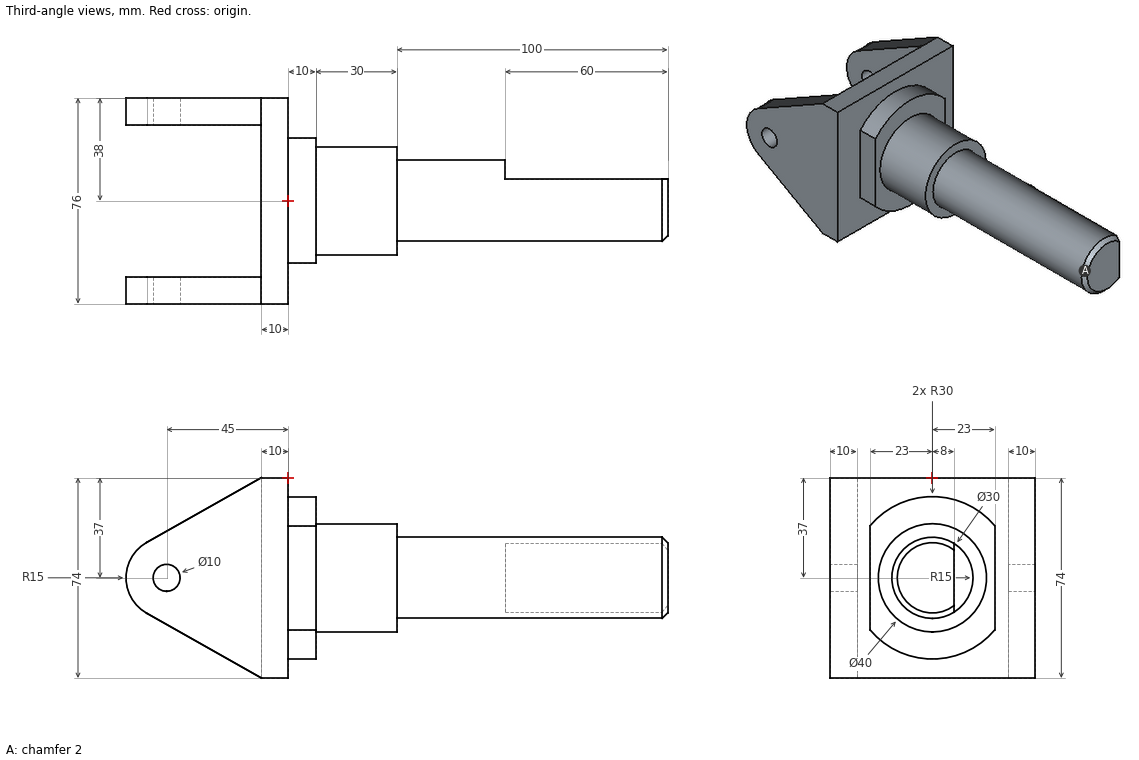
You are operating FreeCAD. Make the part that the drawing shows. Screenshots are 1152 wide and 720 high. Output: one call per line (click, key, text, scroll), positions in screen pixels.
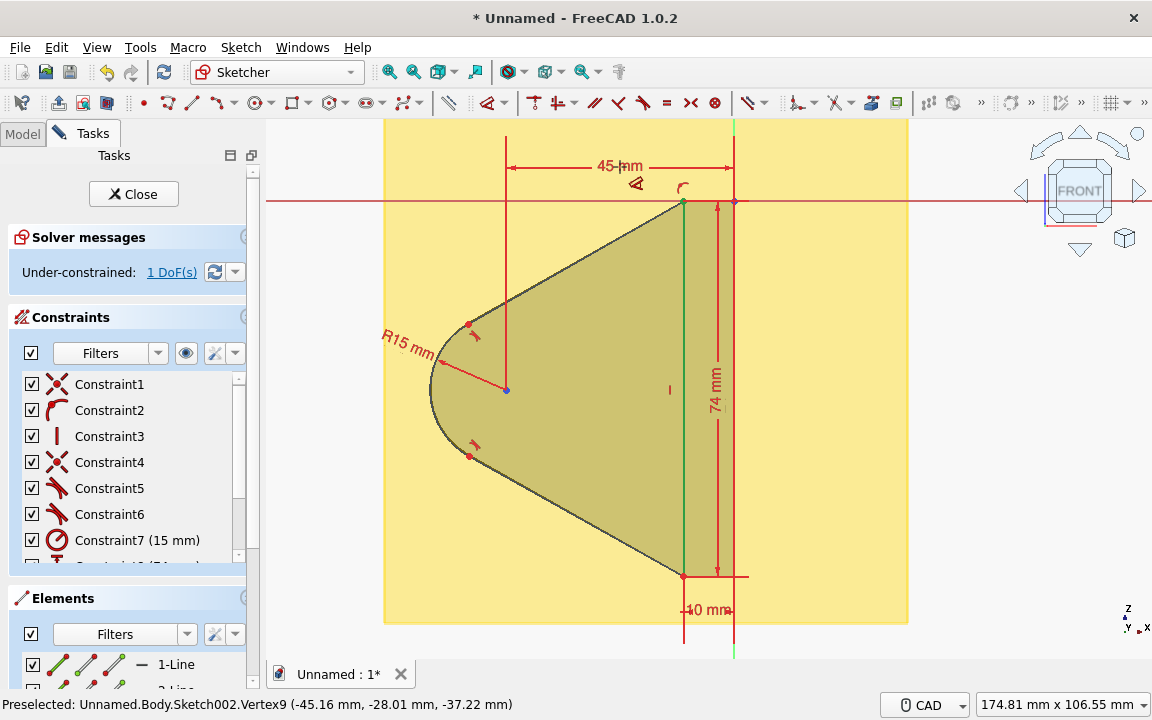
click(506, 390)
click(768, 296)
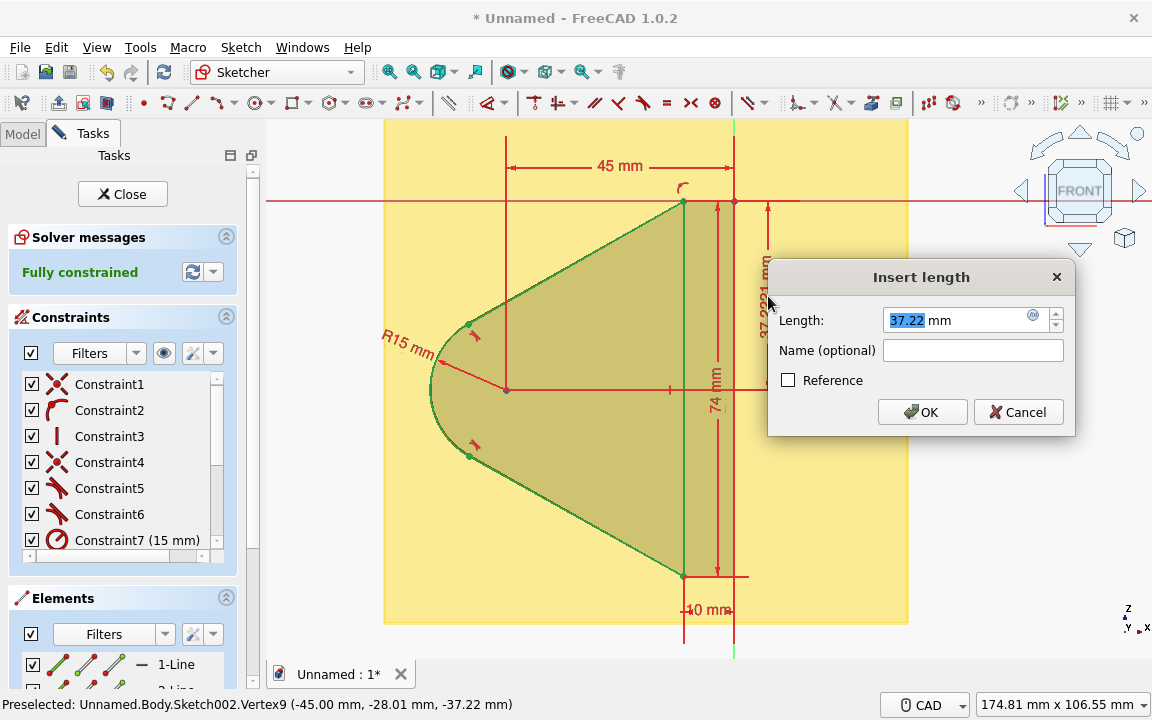
text(37)
key(Return)
key(Escape)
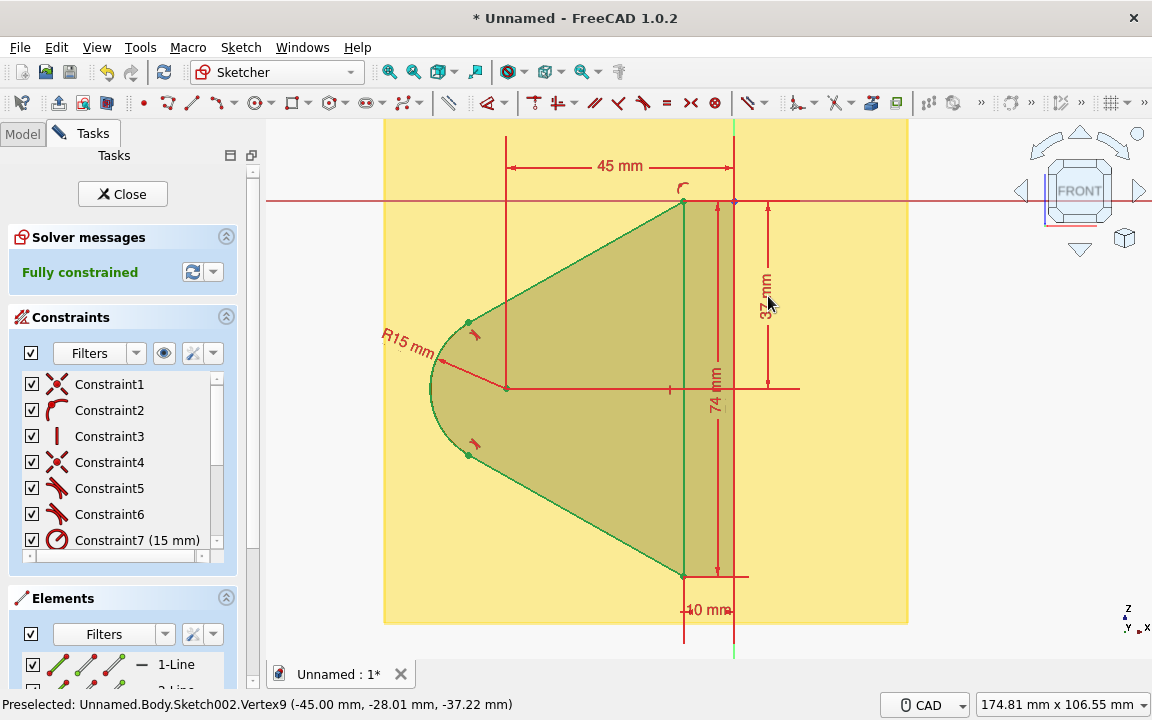
click(123, 194)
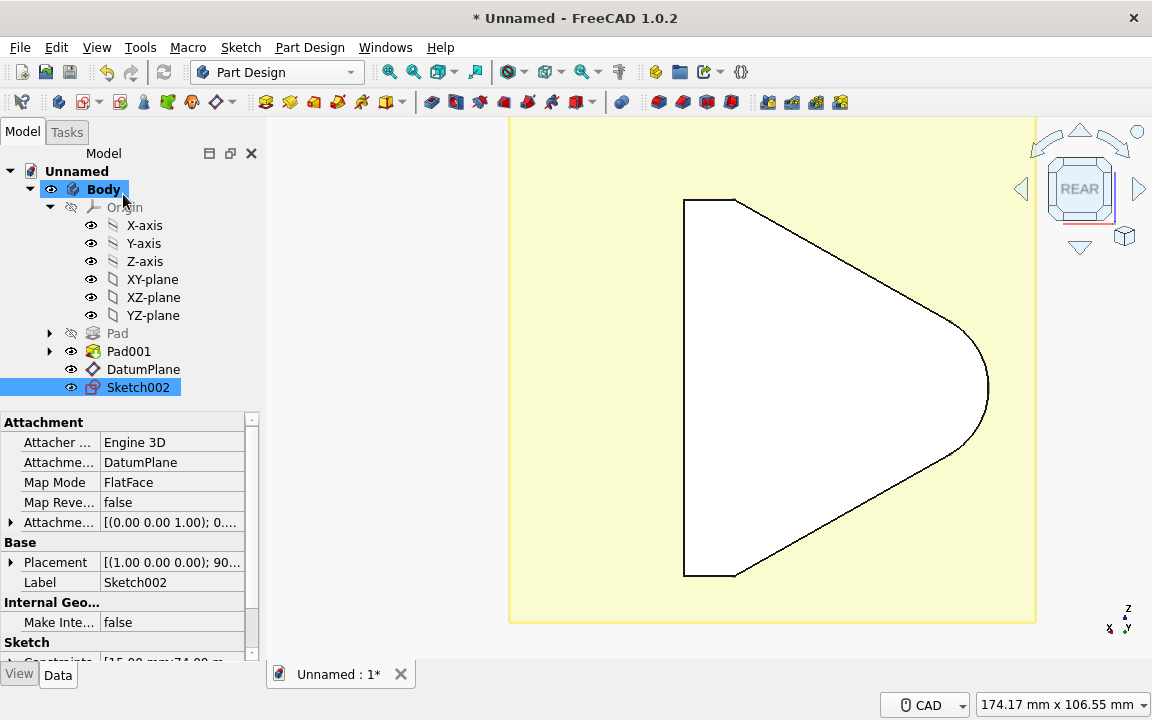
click(266, 102)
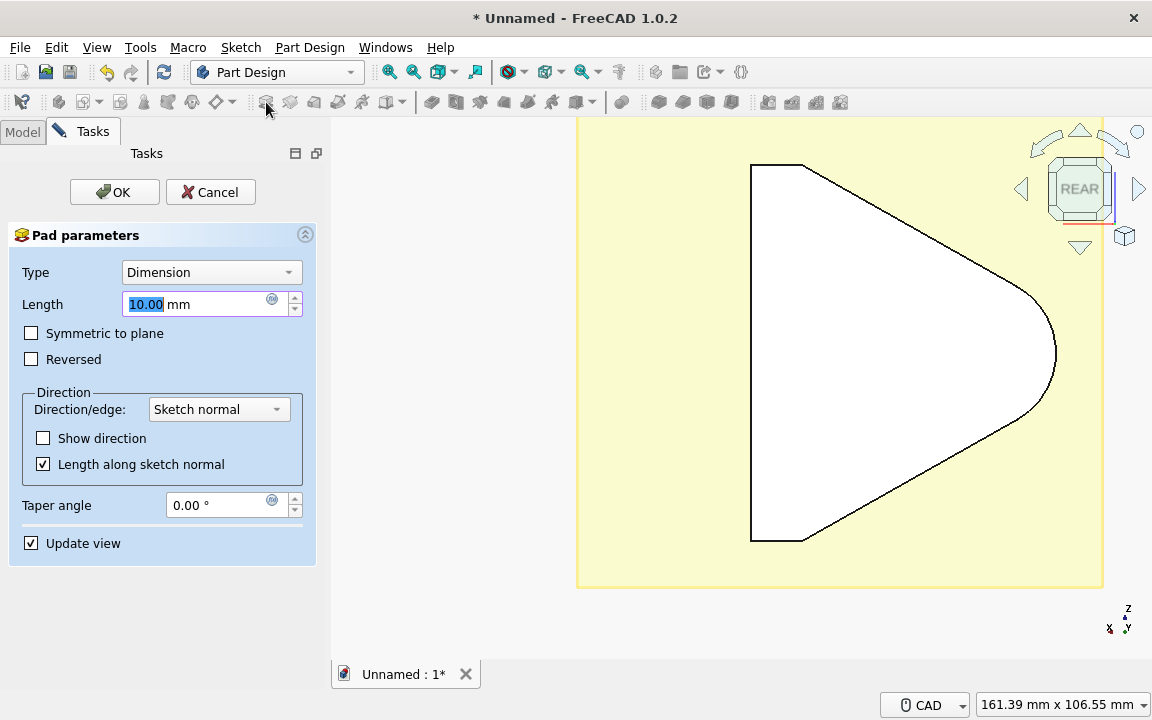
text(10)
key(Tab)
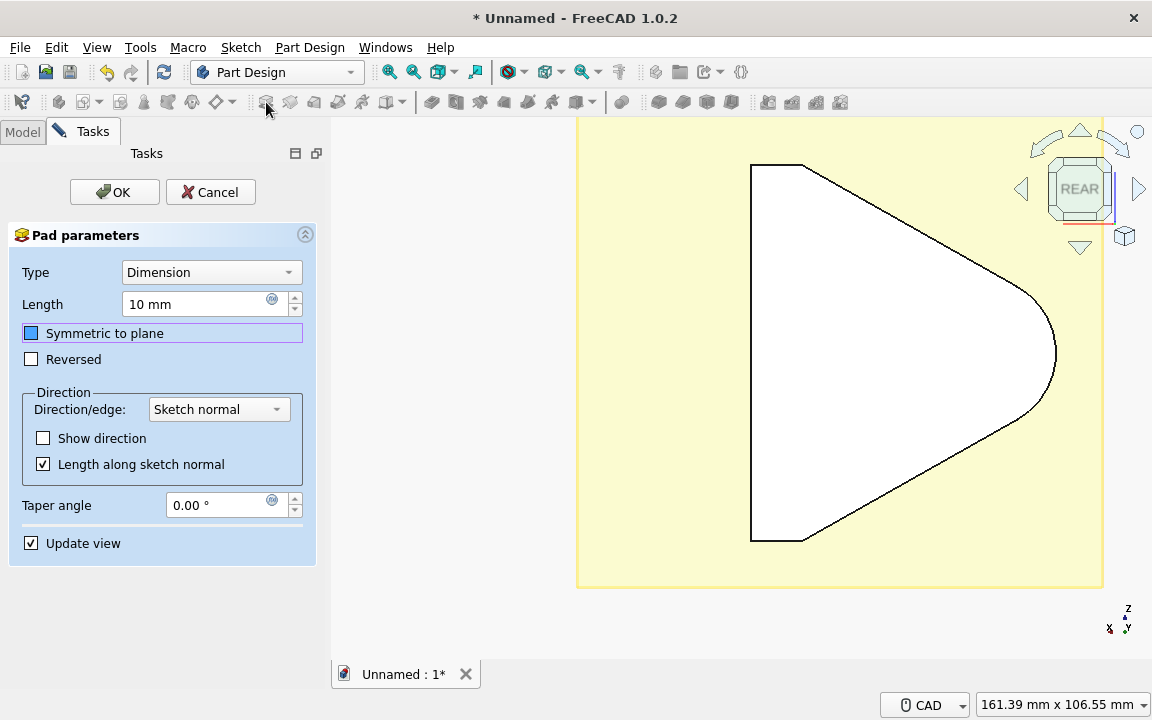
click(115, 192)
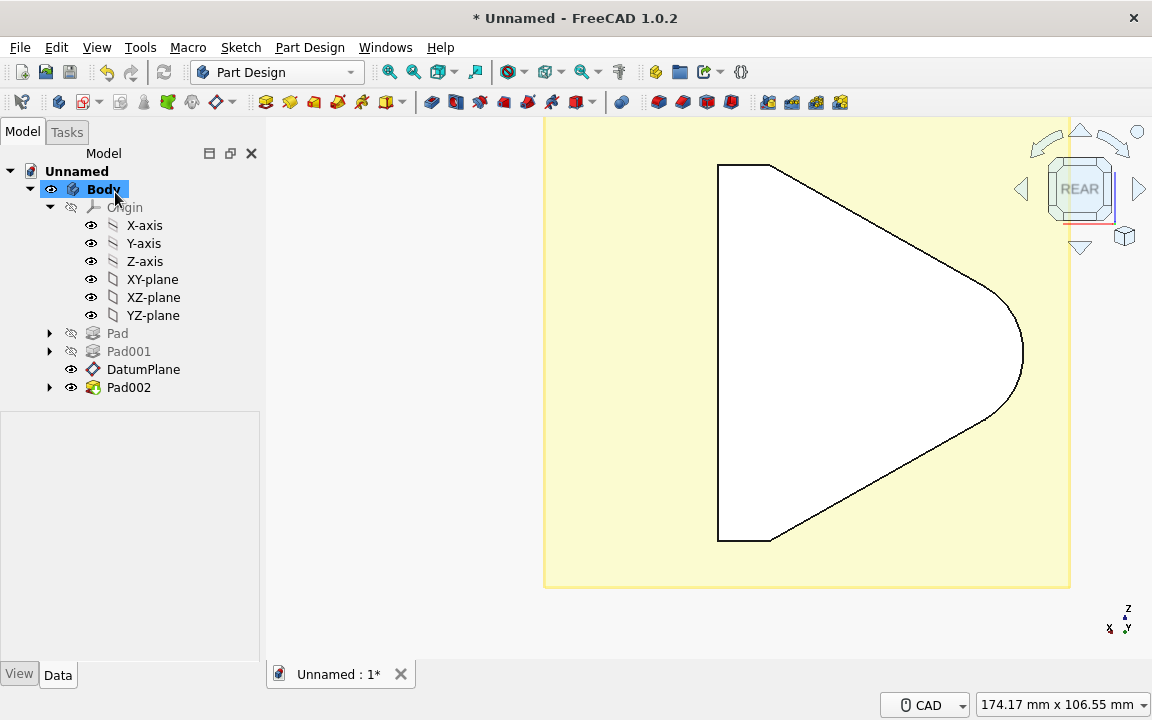
click(116, 369)
key(space)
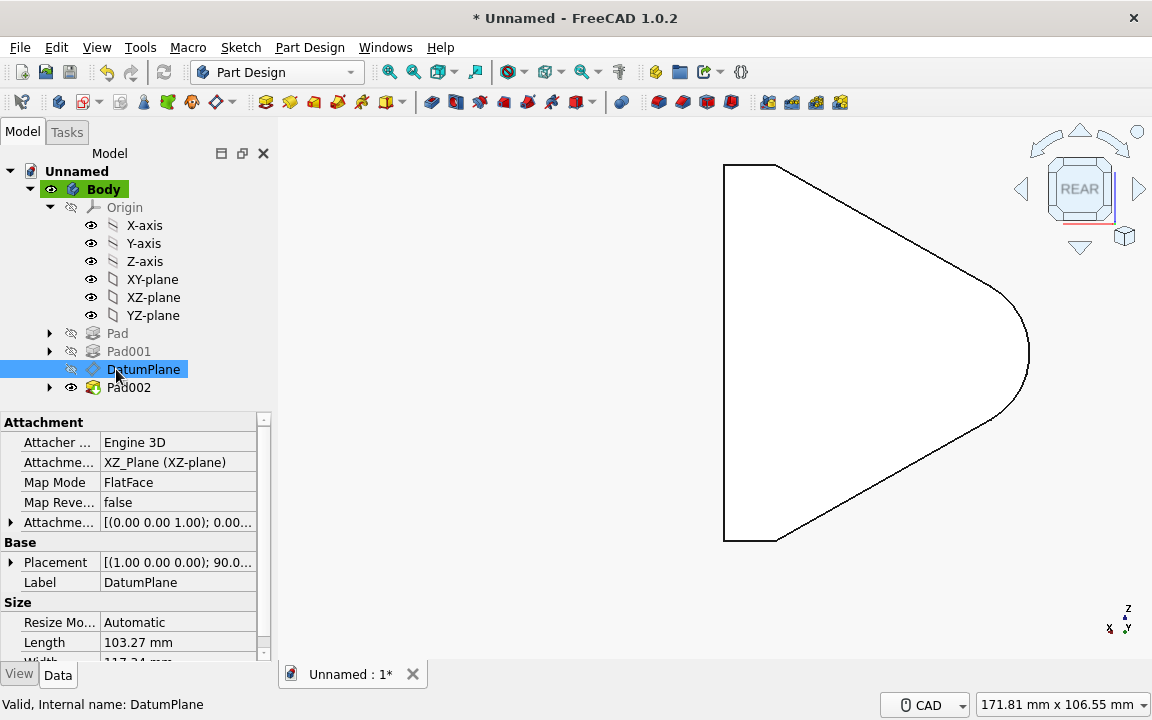
key(0)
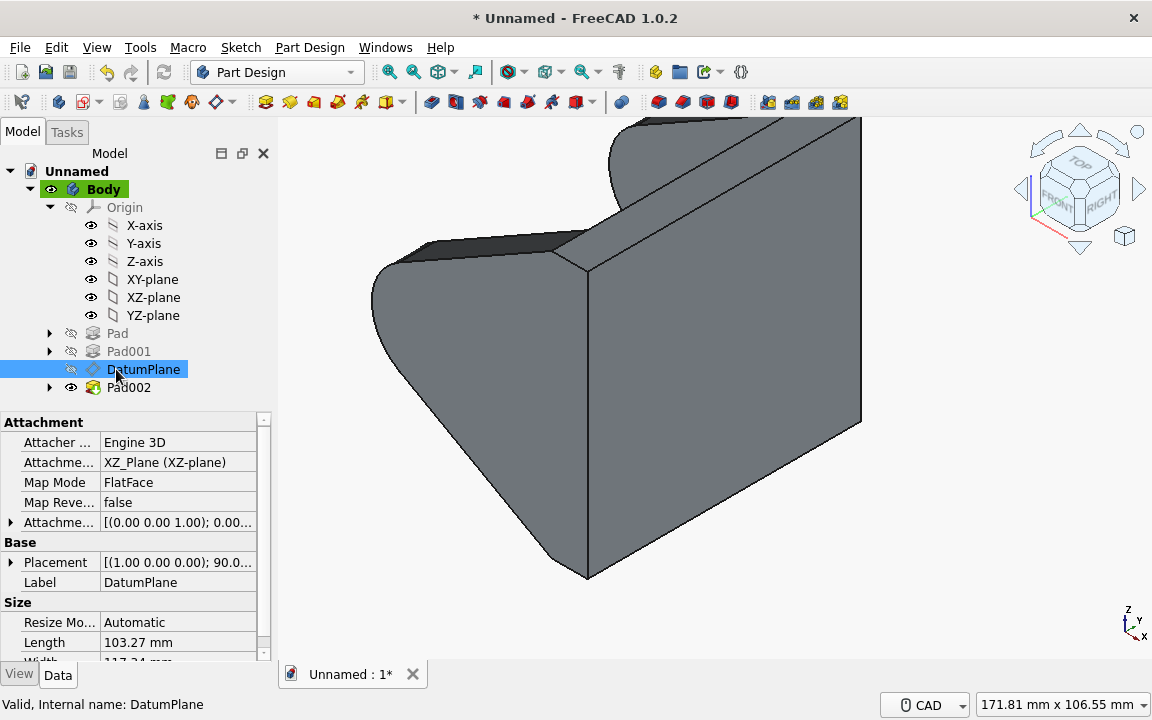
click(390, 72)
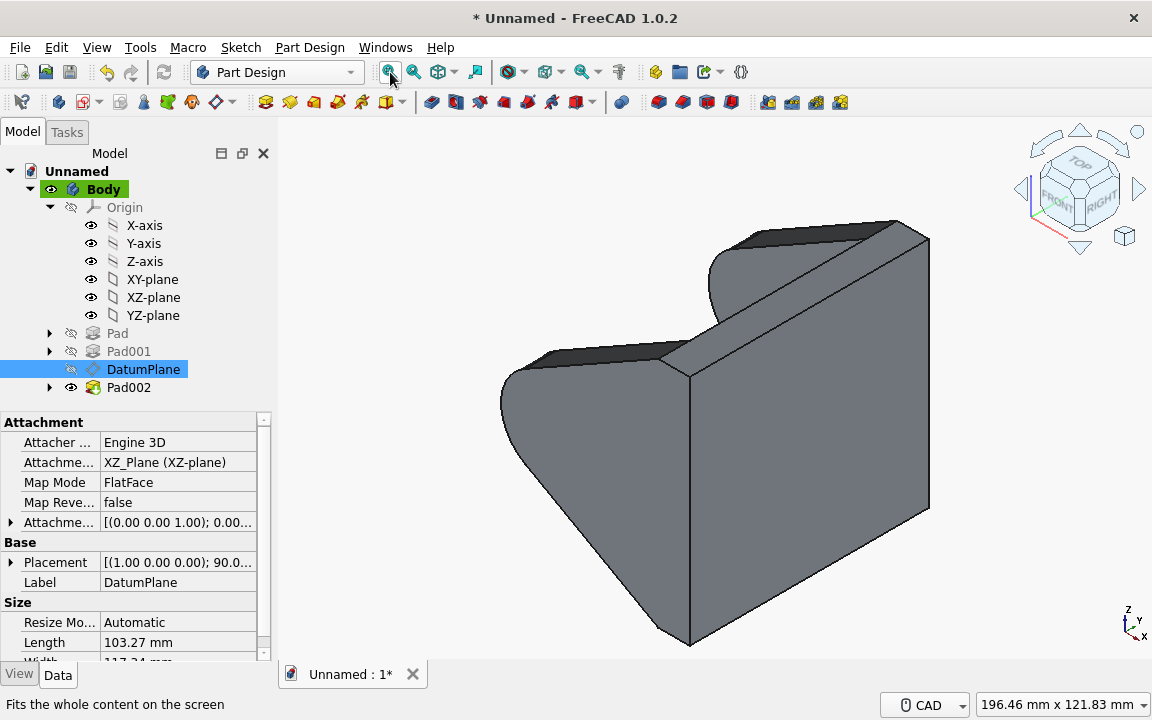
click(595, 456)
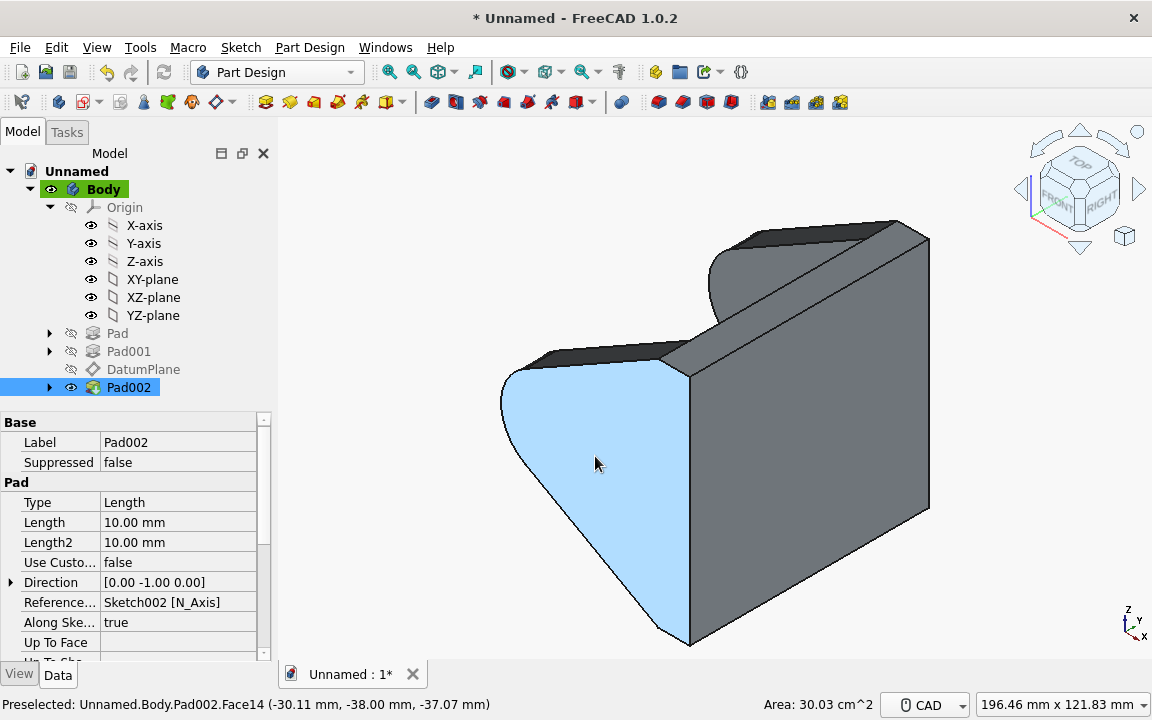
click(84, 102)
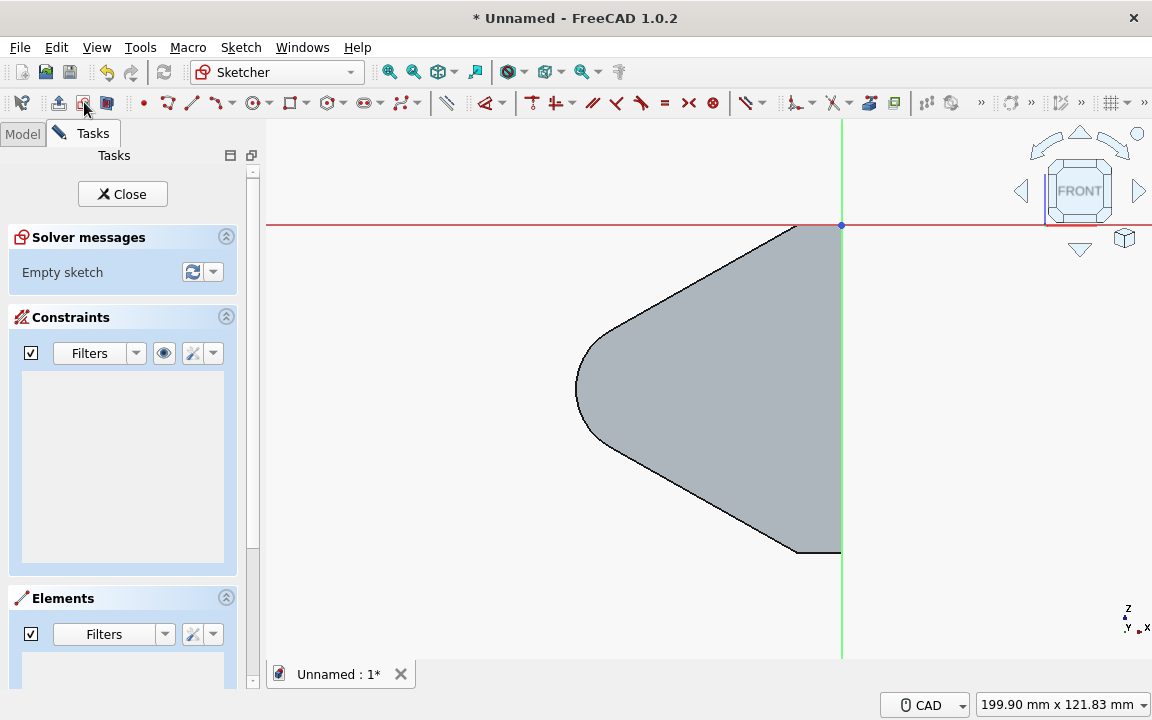
scroll(643, 389, up, 10)